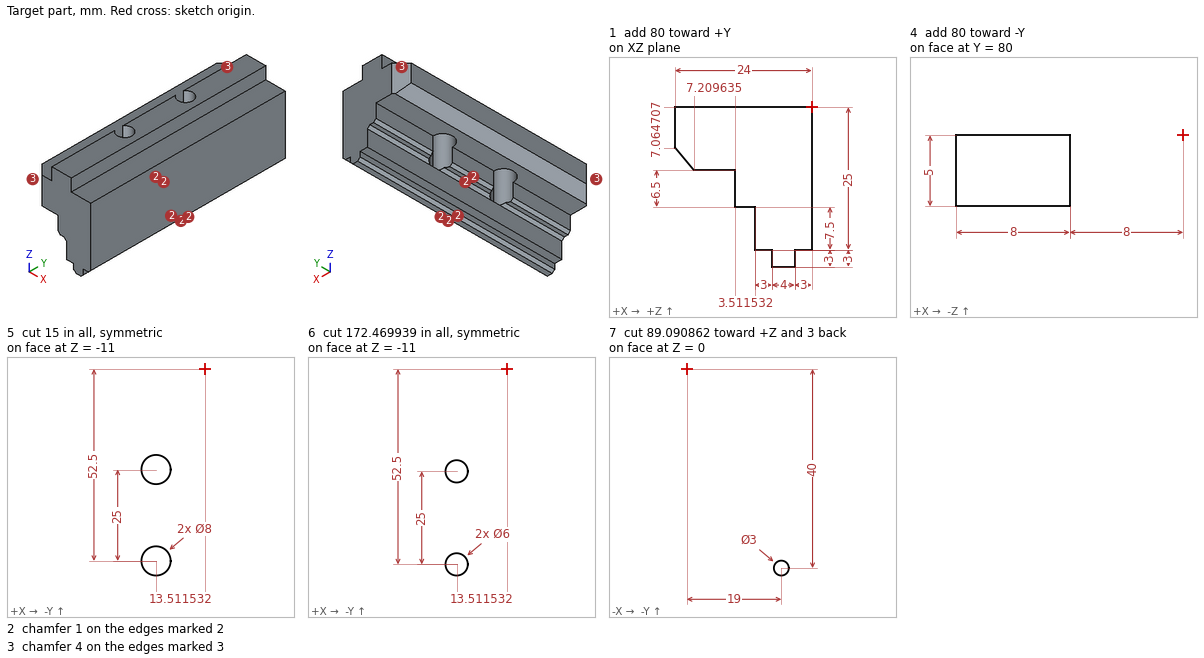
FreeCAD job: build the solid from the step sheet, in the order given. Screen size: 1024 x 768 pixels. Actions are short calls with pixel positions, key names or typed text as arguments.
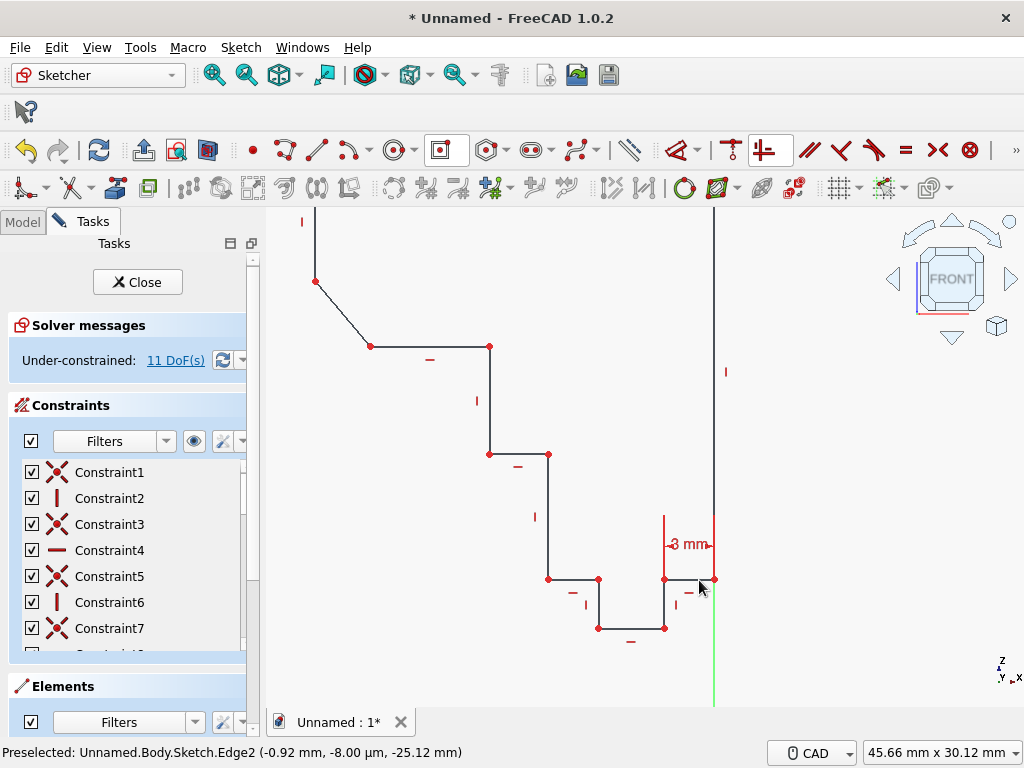
click(664, 594)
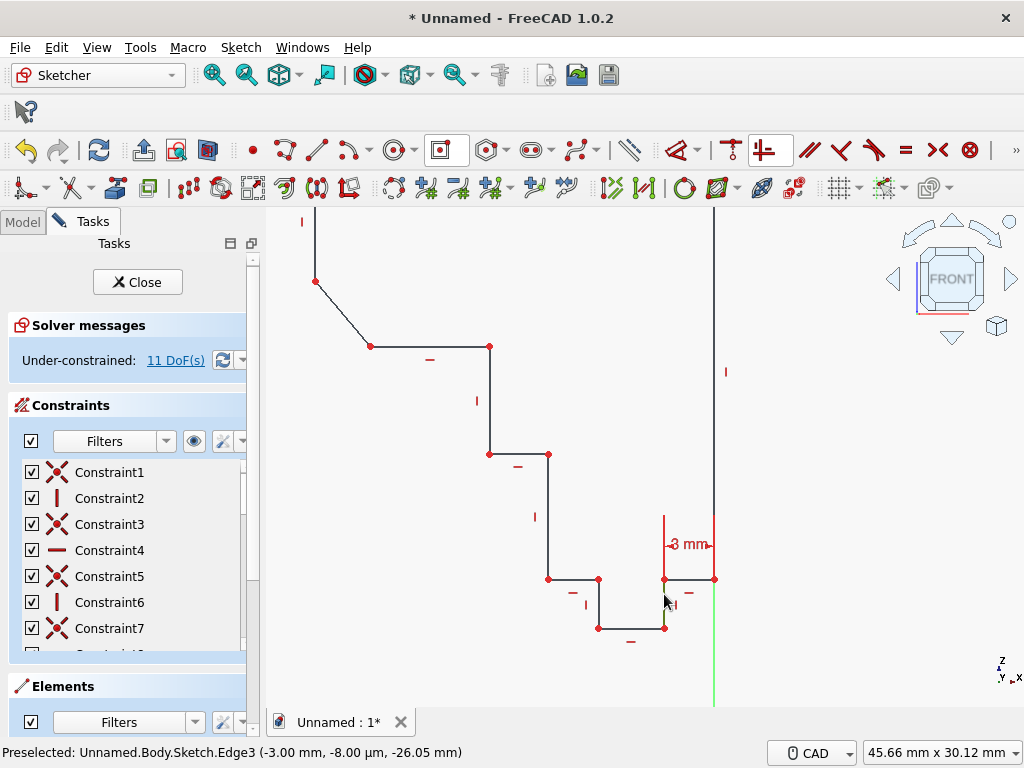
key(i)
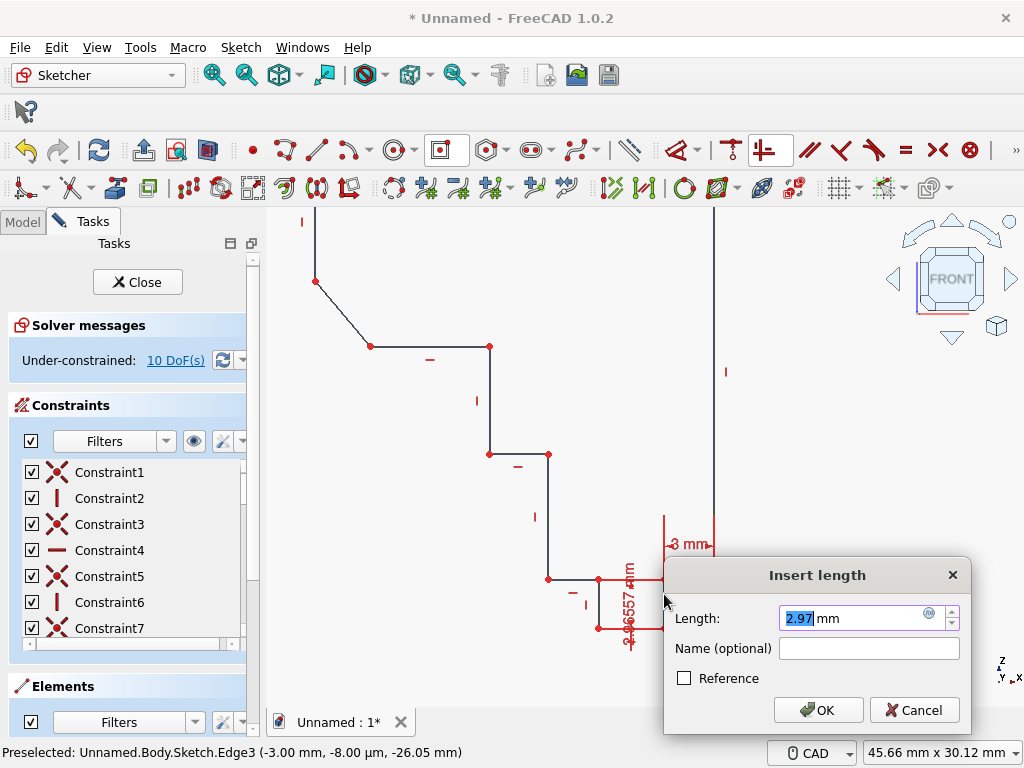
text(3)
key(Return)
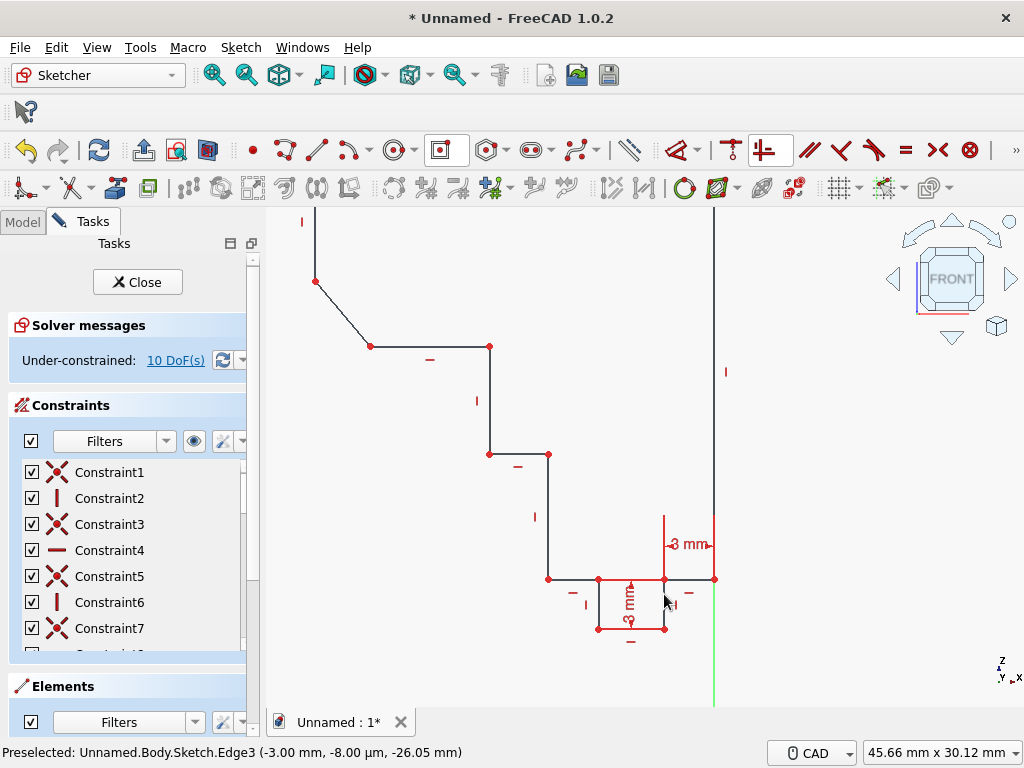
click(645, 629)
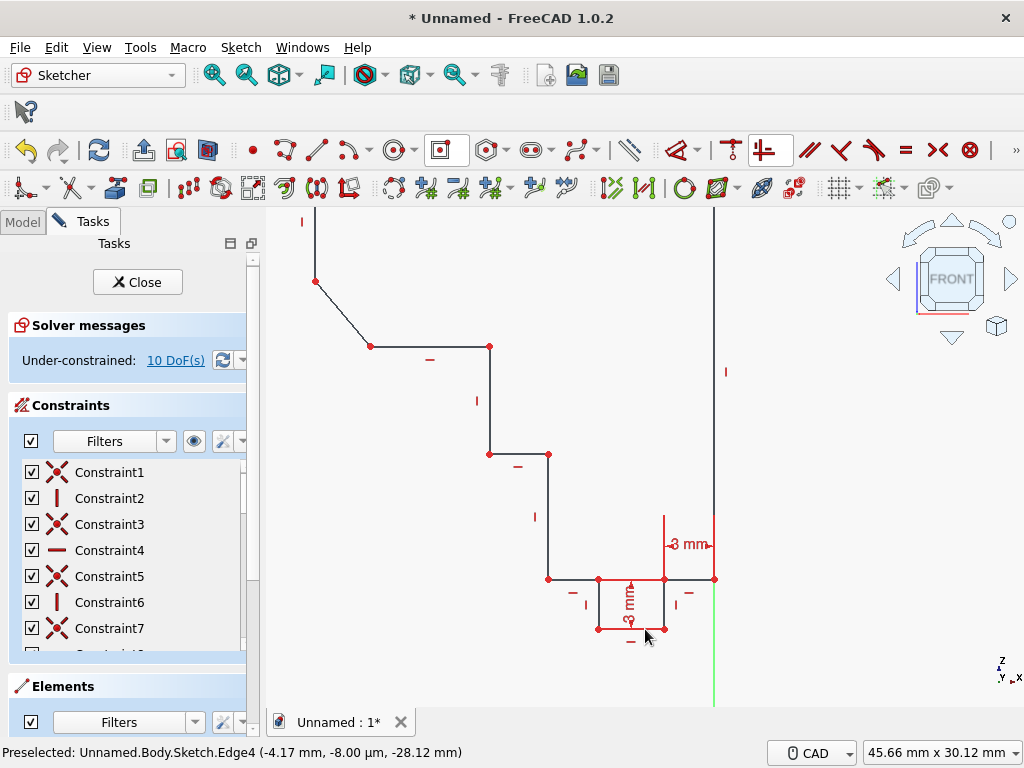
key(l)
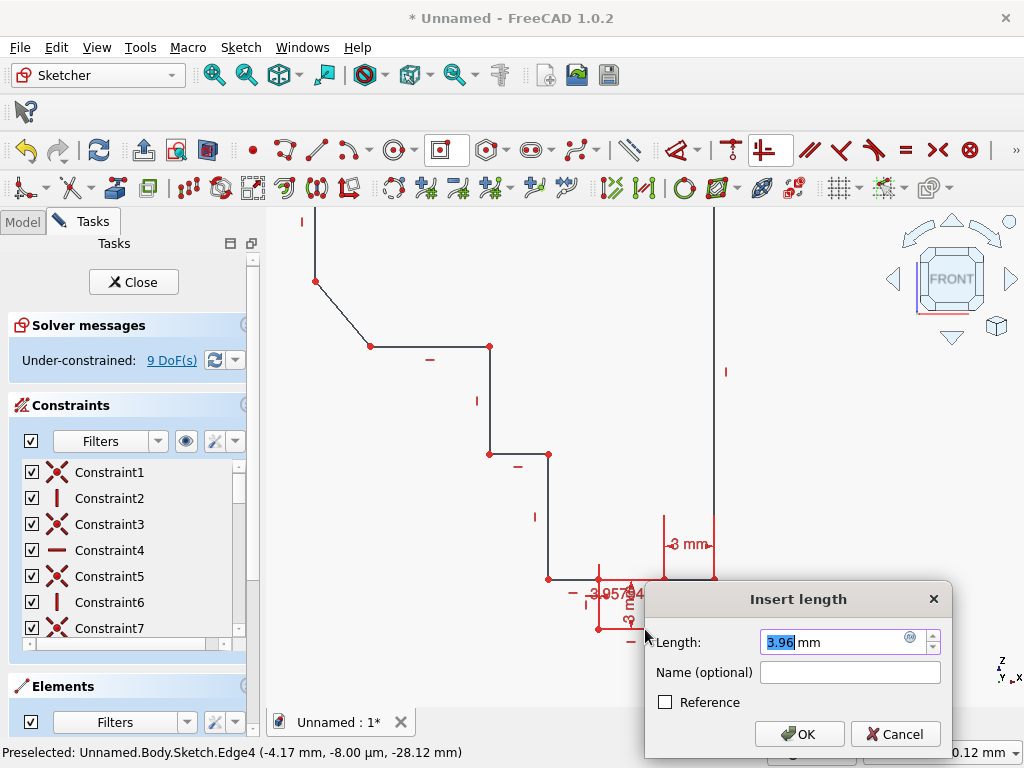
text(4)
key(Return)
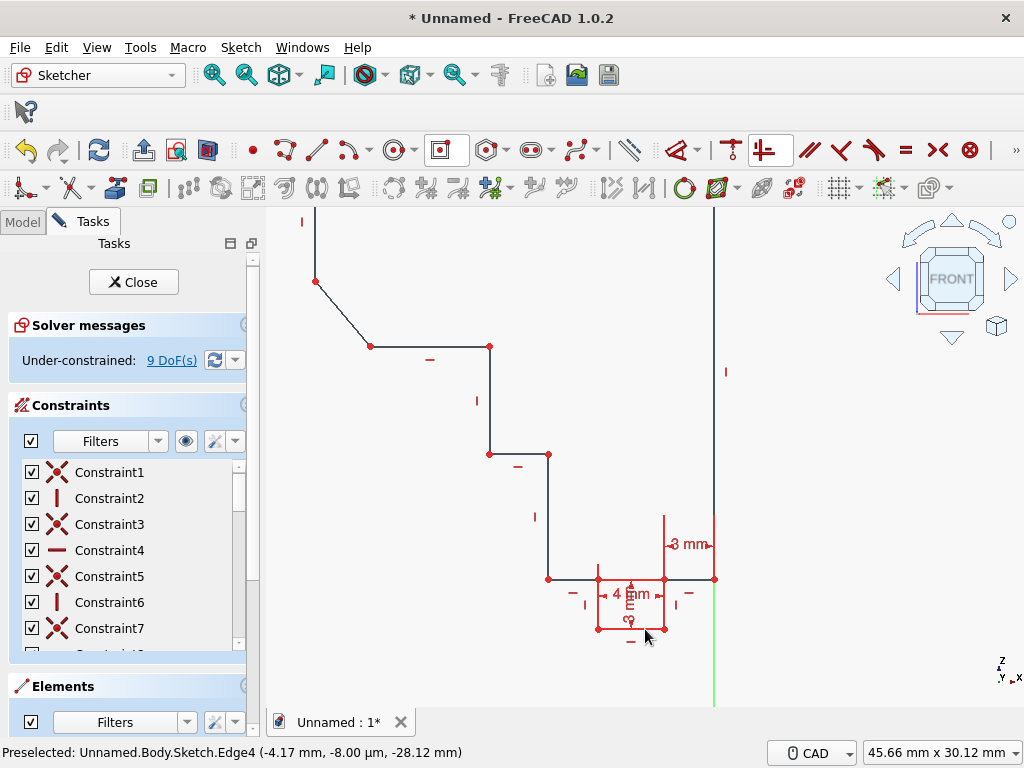
click(598, 614)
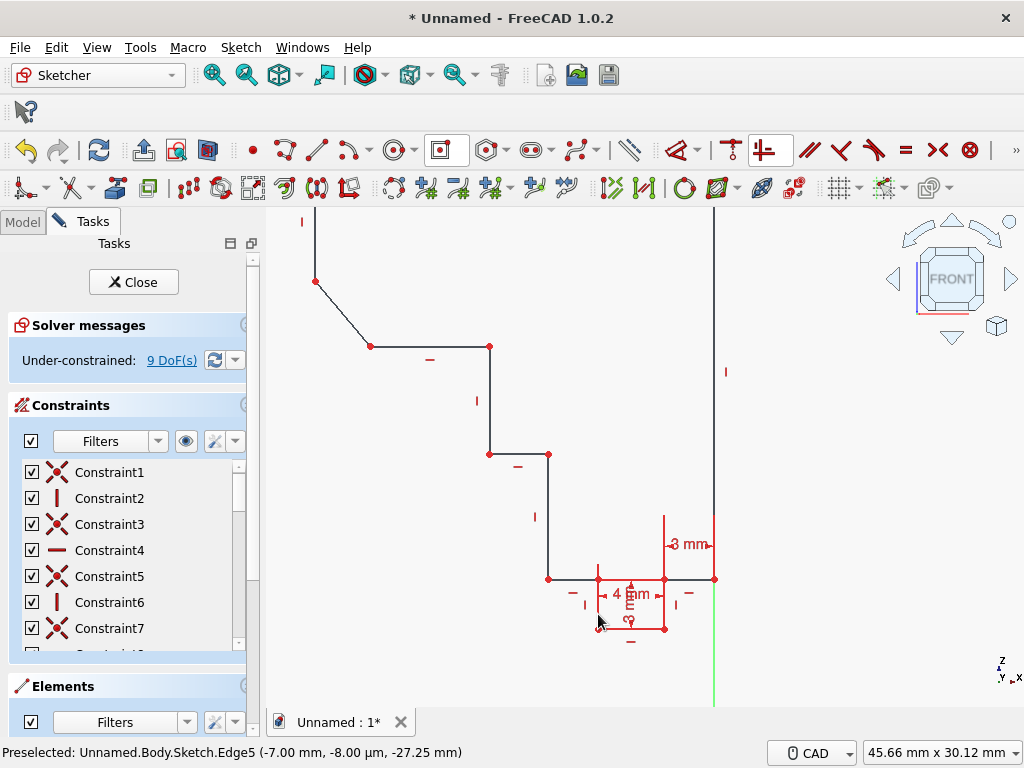
click(700, 150)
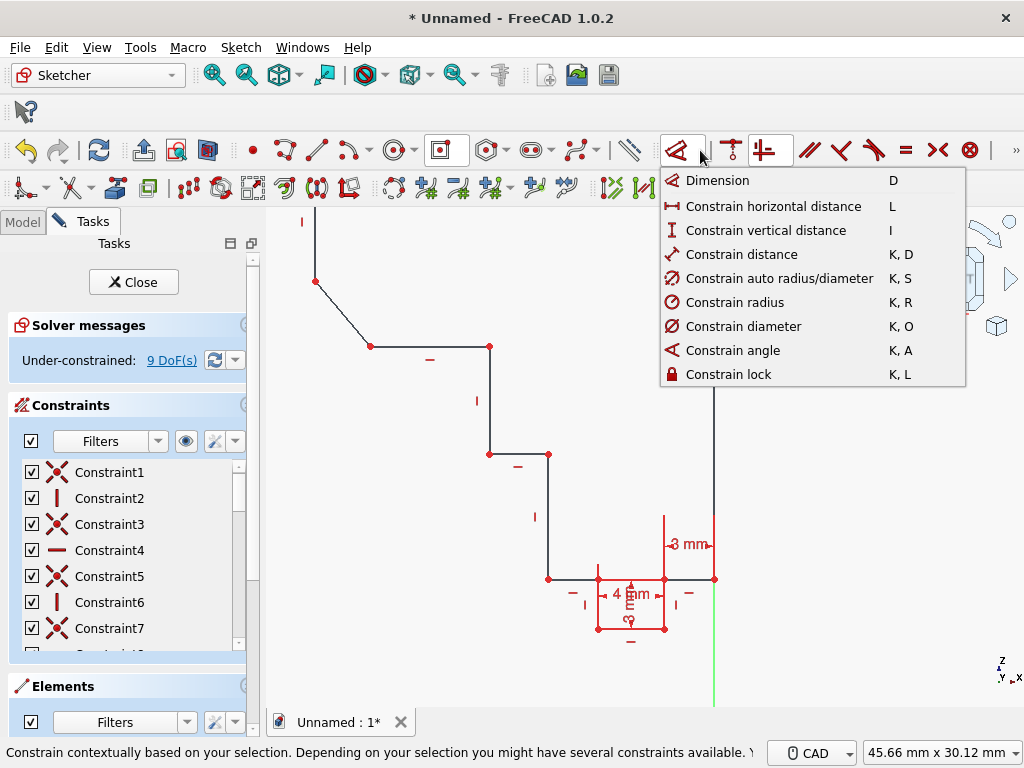
click(813, 230)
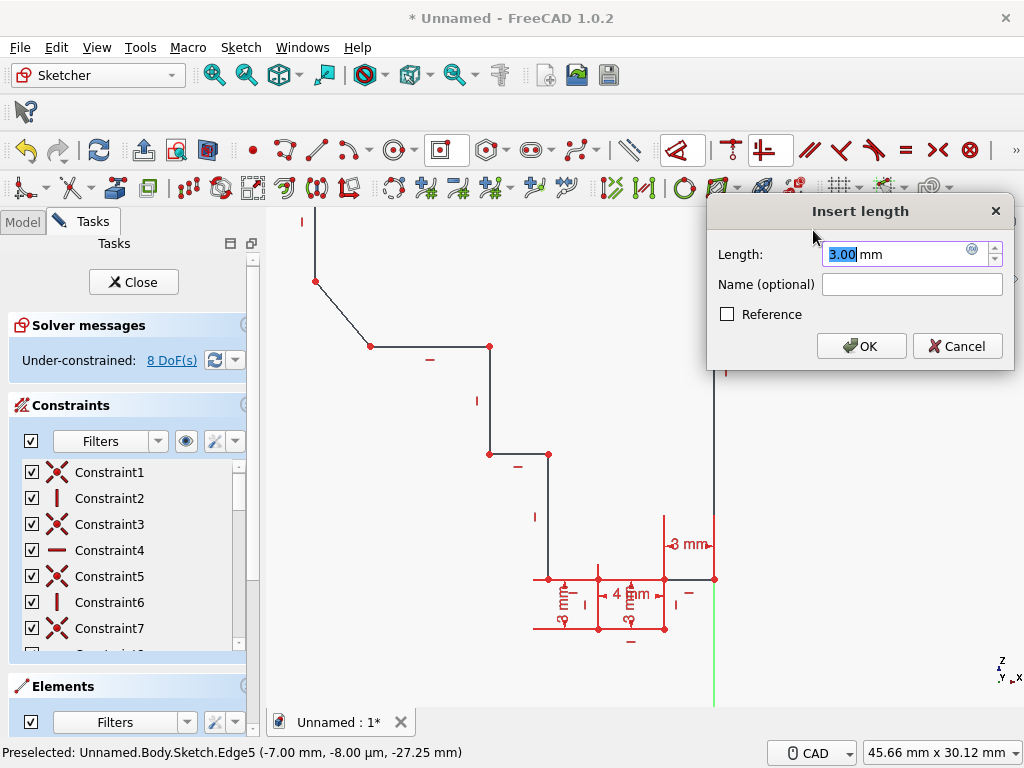
text(3)
key(Return)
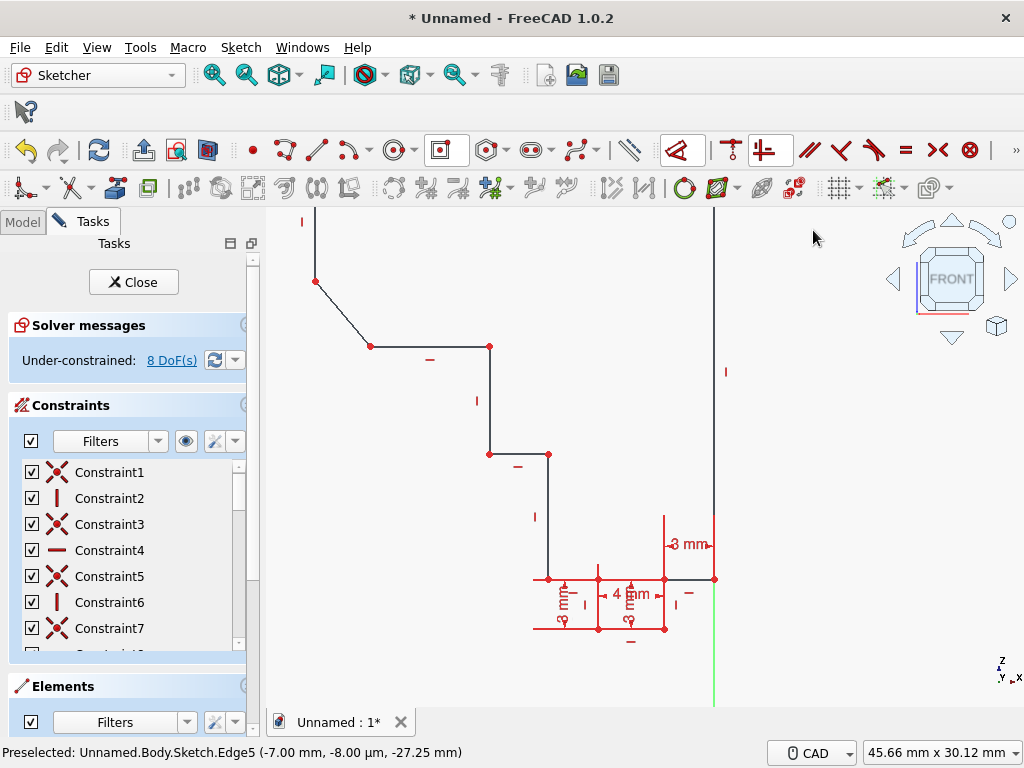
click(583, 580)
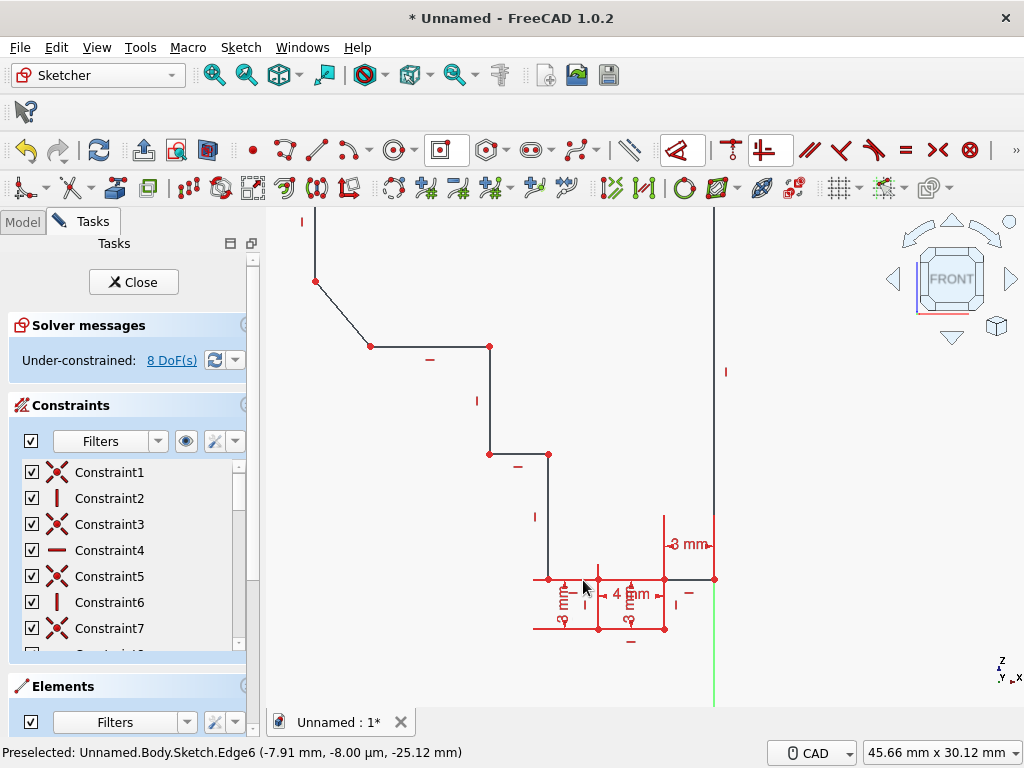
key(l)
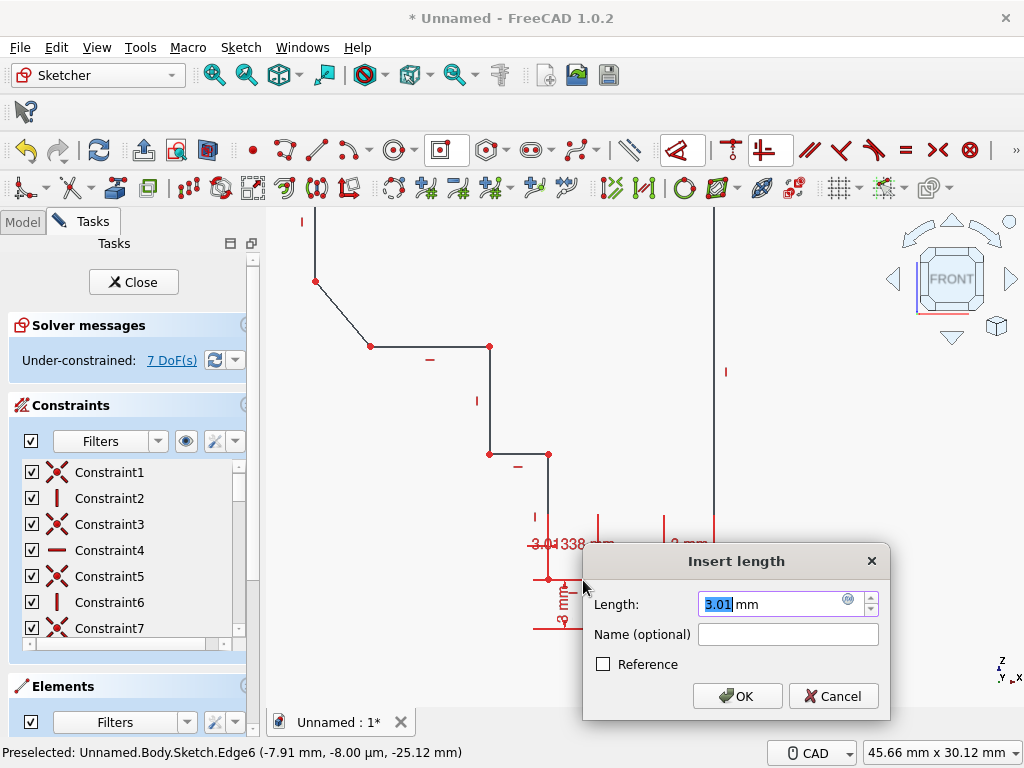
text(3)
key(Return)